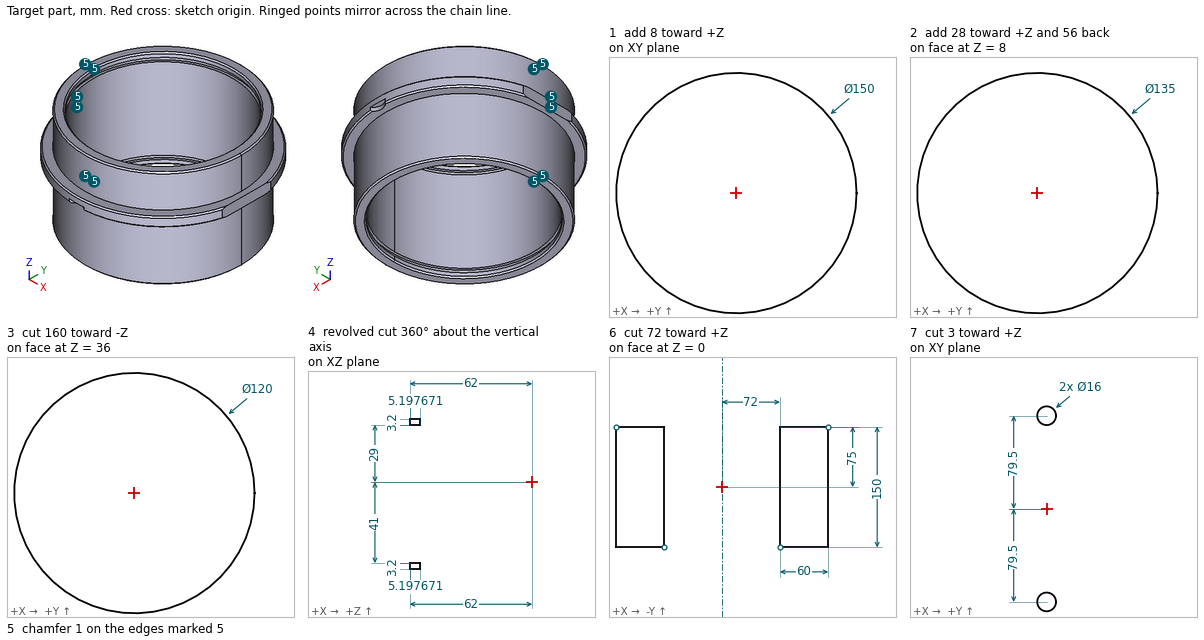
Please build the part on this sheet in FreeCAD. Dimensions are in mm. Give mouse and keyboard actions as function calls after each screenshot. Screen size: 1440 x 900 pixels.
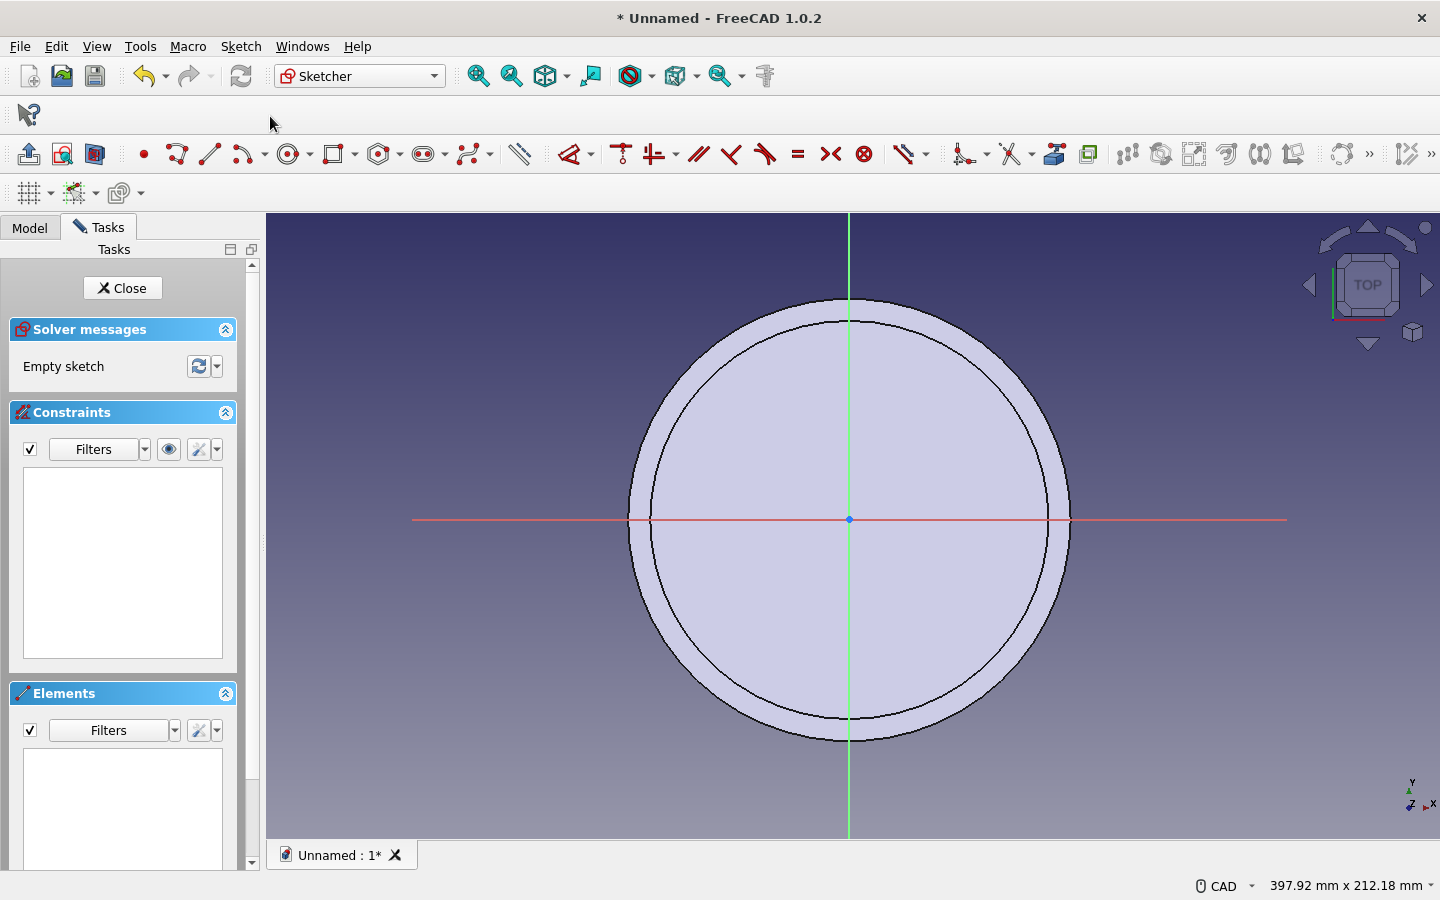
key(g)
key(c)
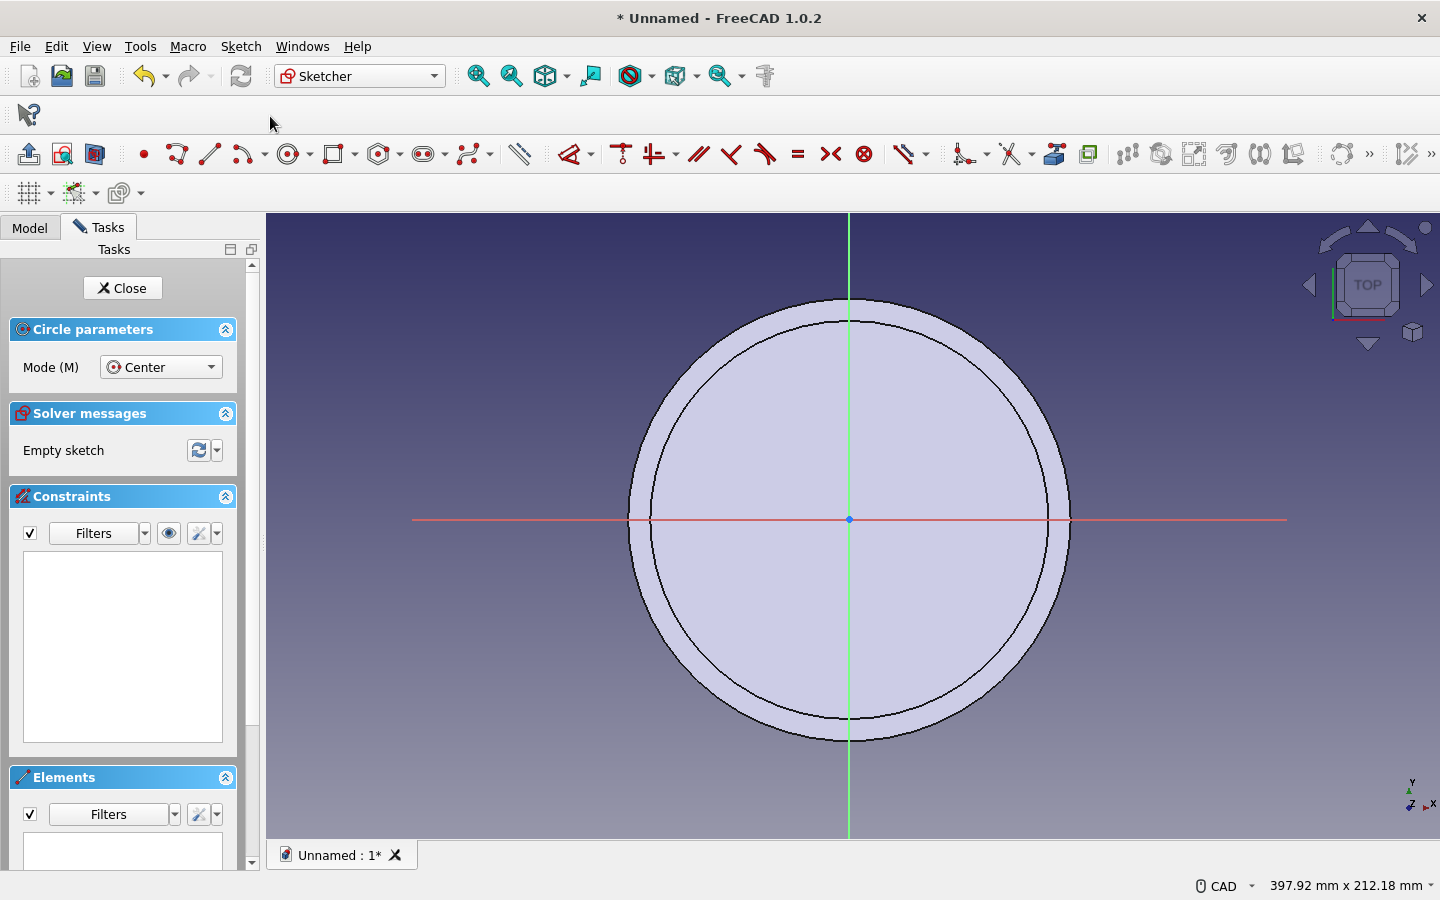
click(849, 520)
click(975, 395)
key(Escape)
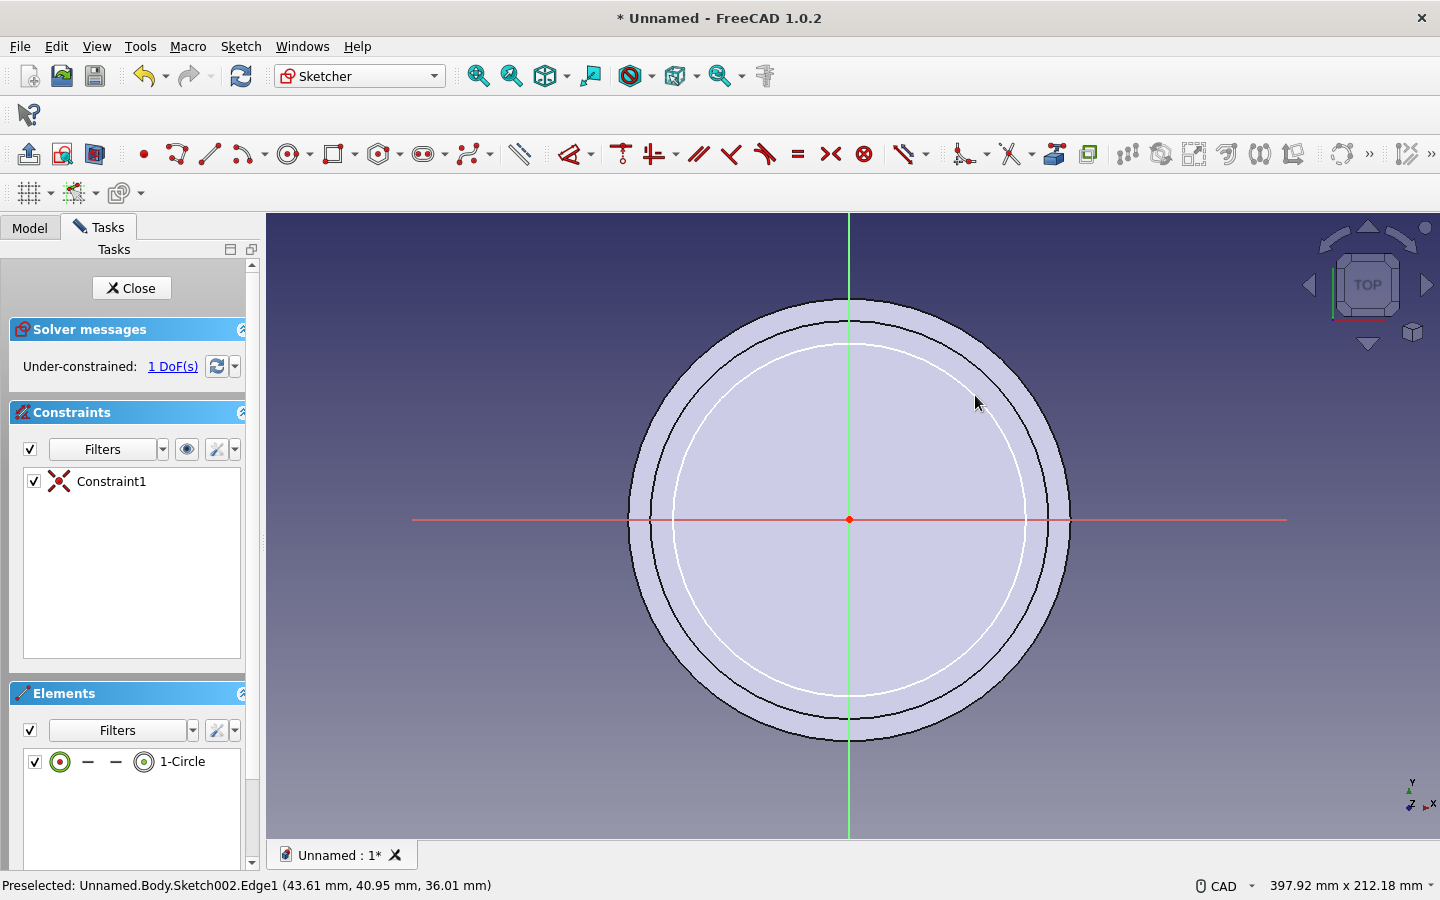
click(568, 154)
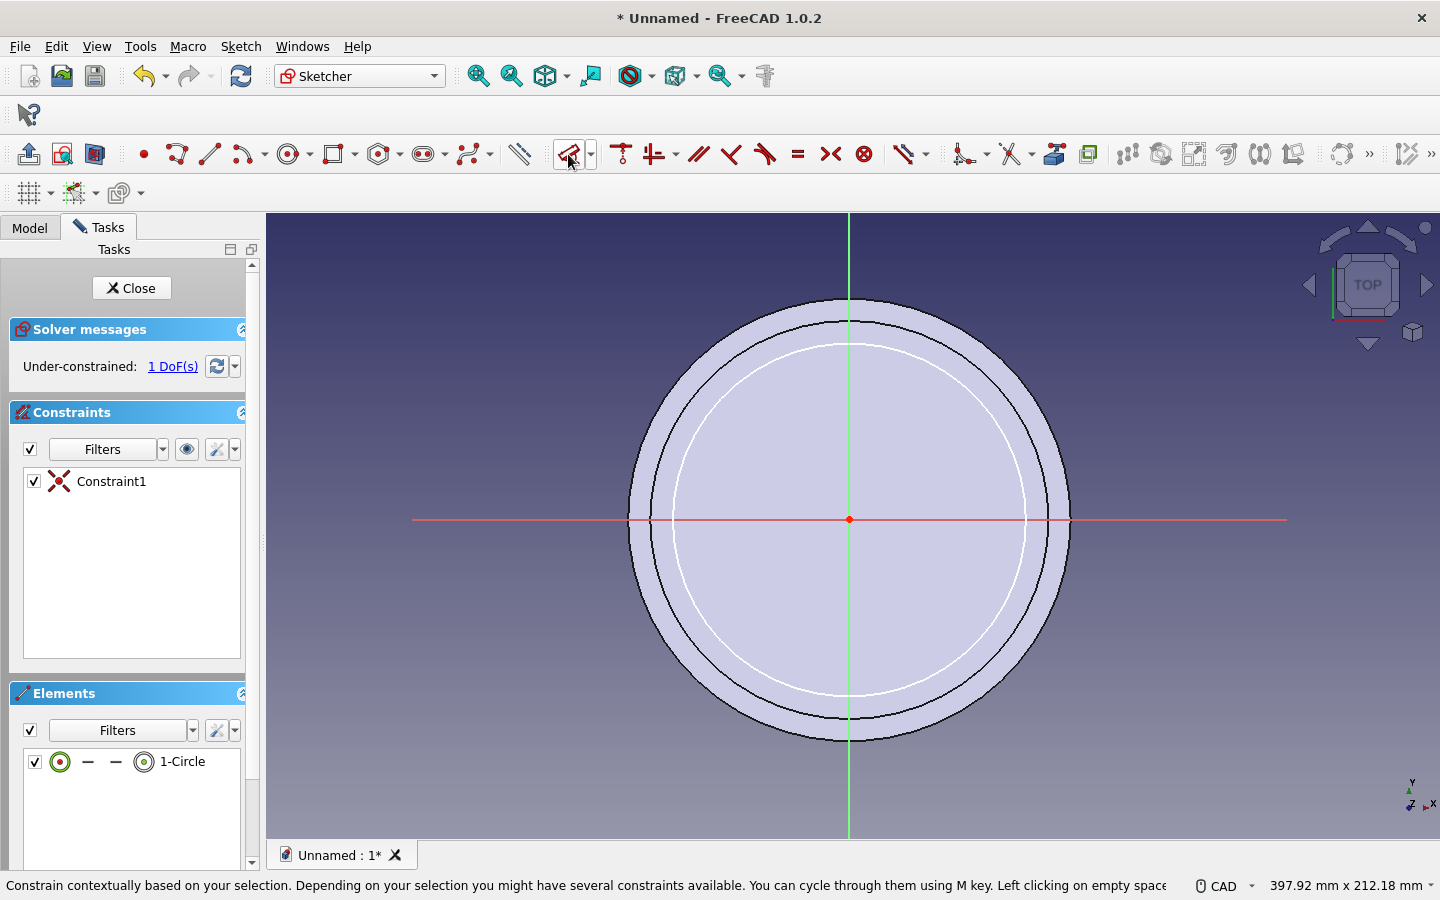
click(974, 395)
click(997, 372)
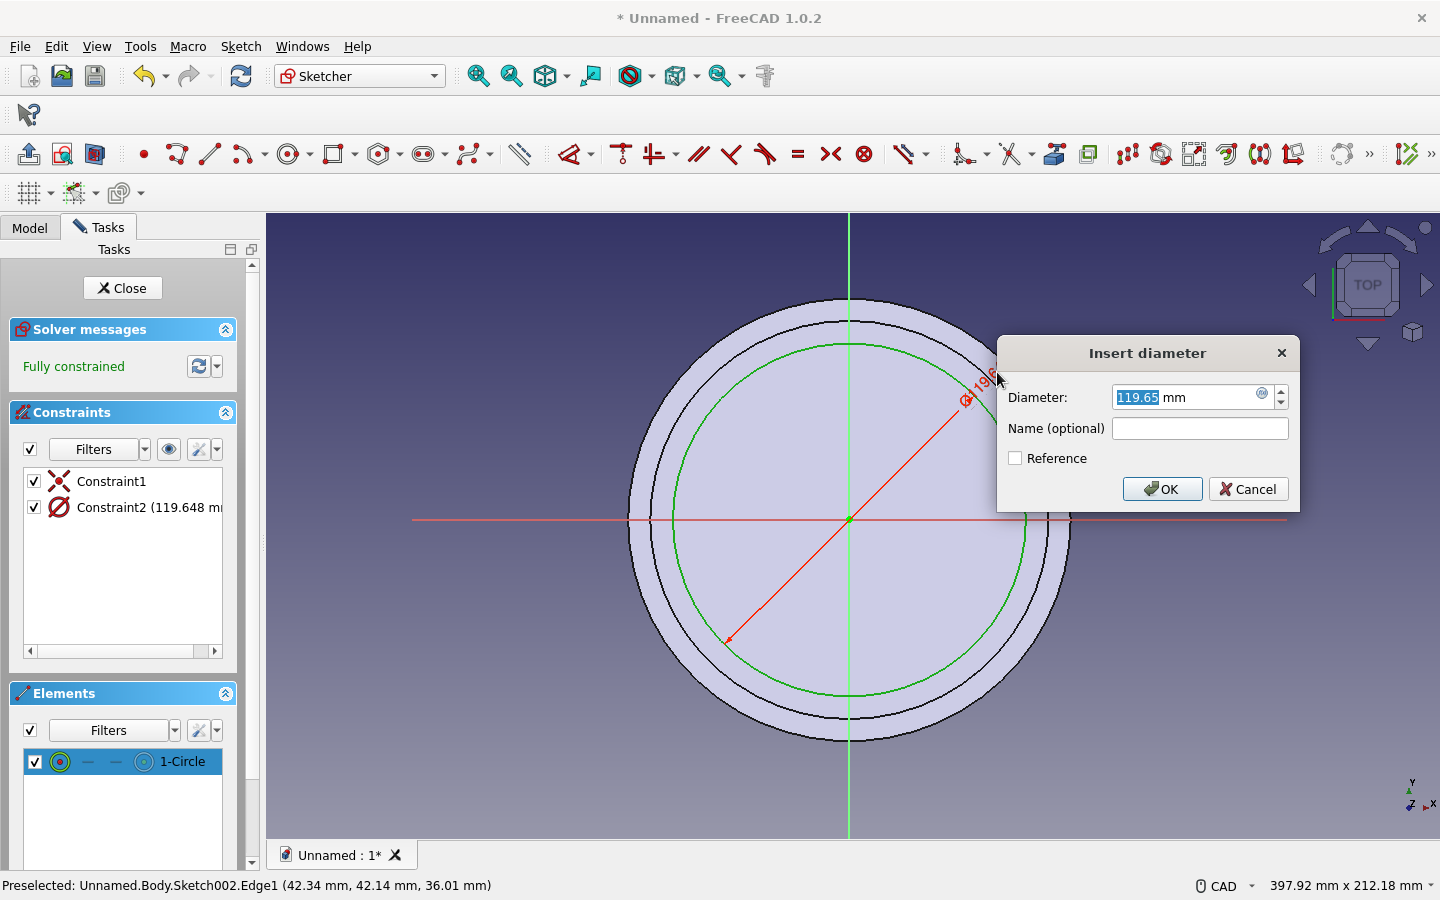
text(120)
key(Return)
key(Escape)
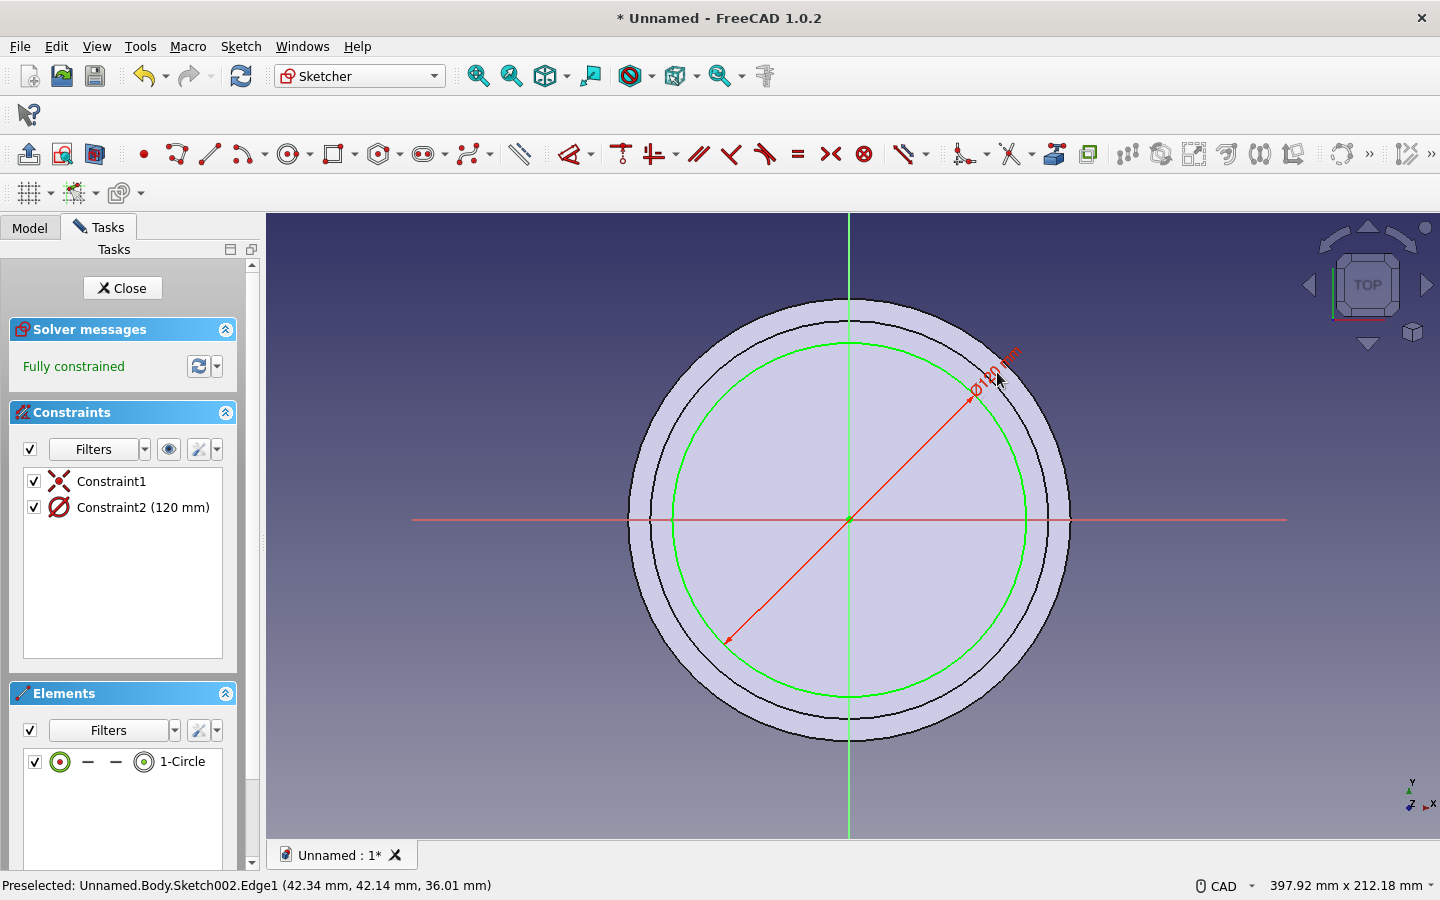
click(123, 288)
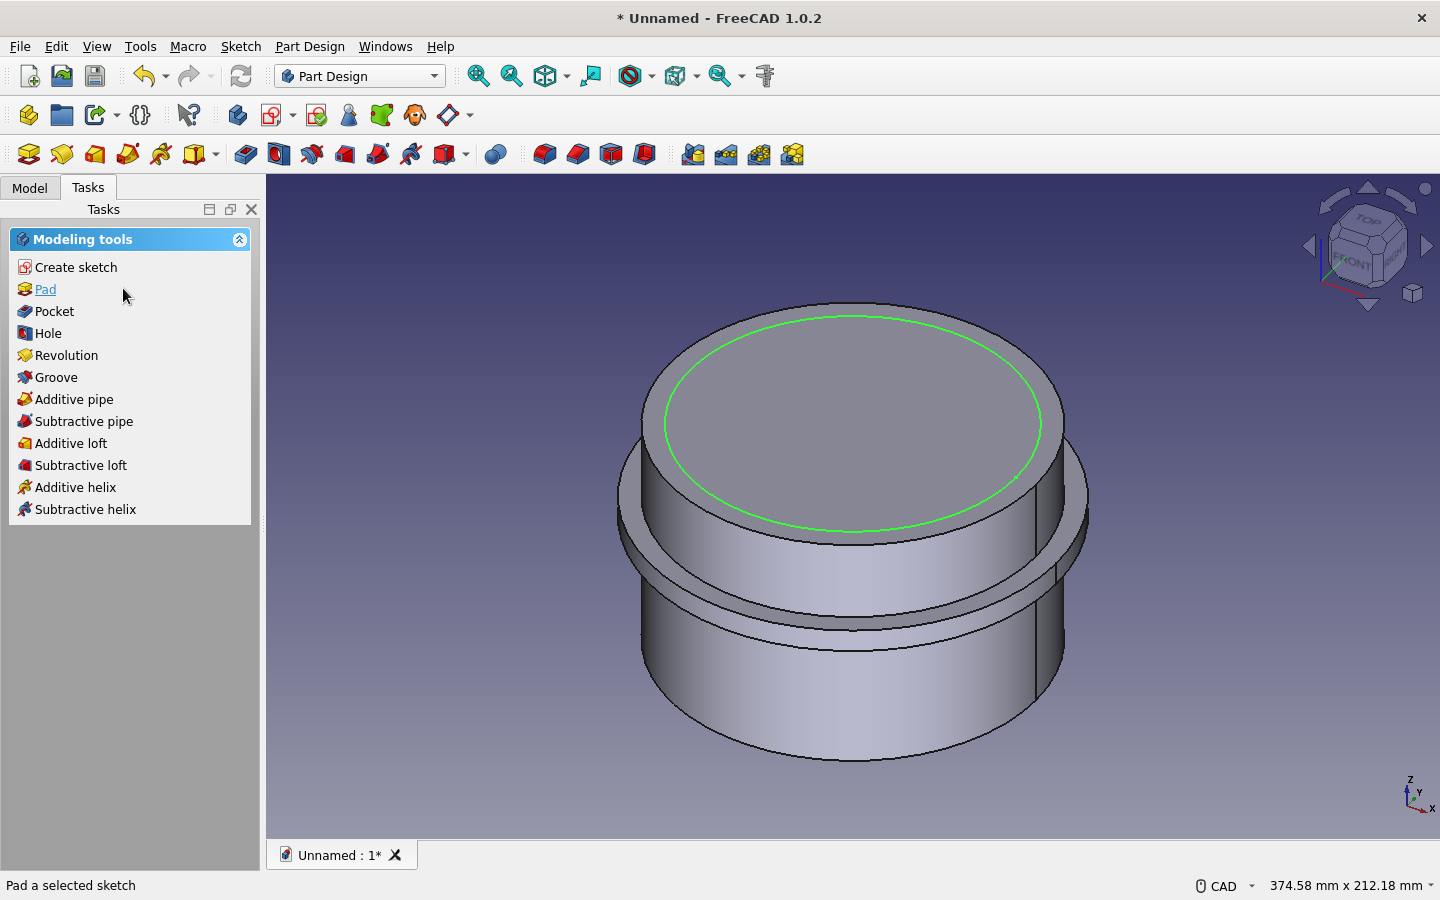
click(246, 154)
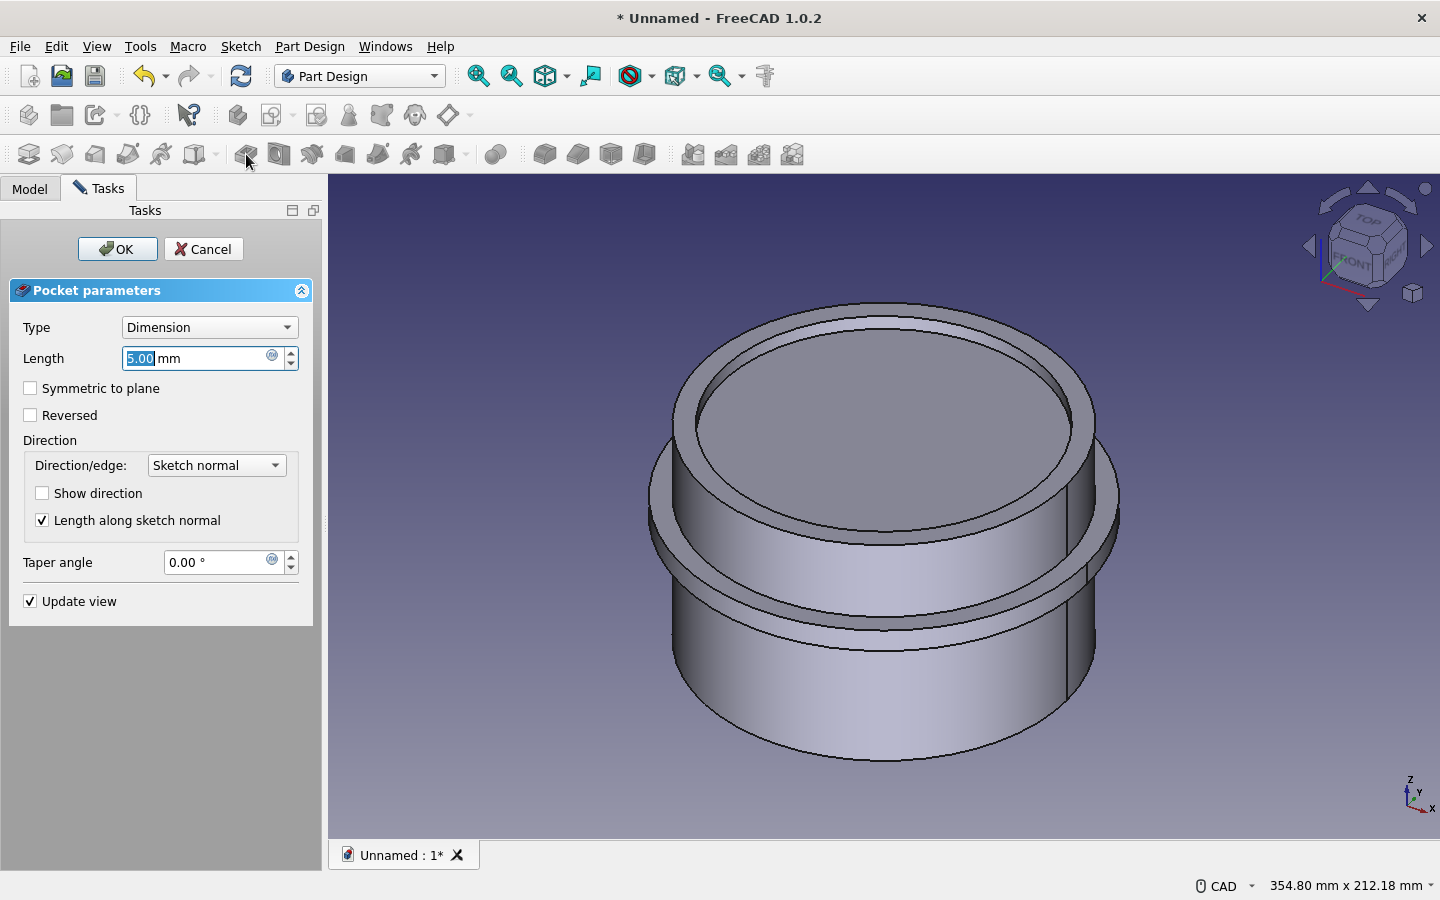
text(160)
key(Tab)